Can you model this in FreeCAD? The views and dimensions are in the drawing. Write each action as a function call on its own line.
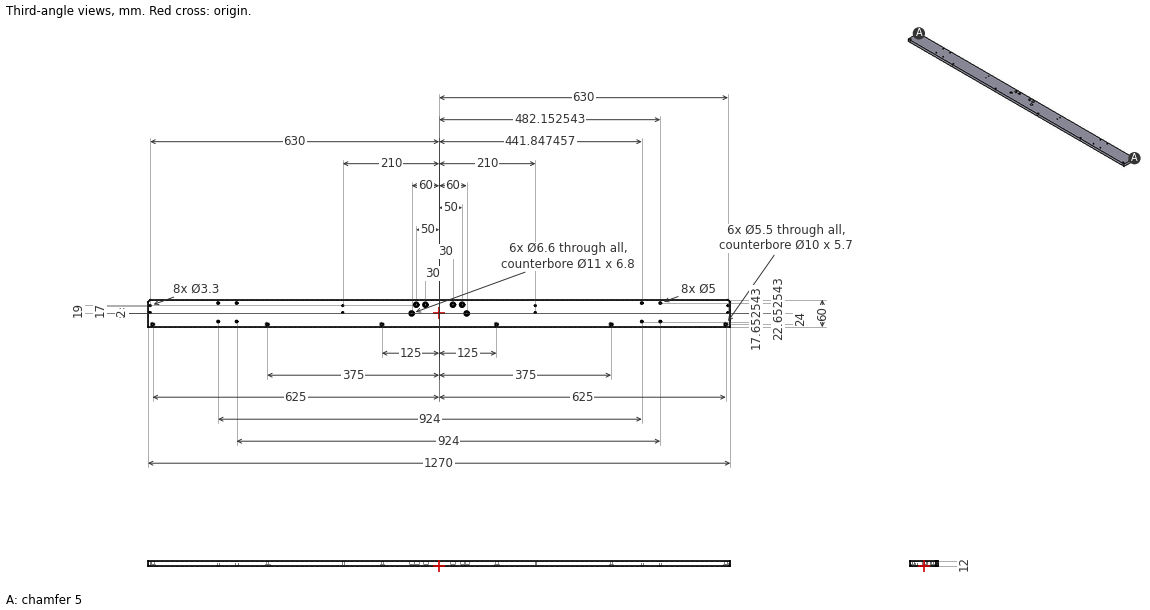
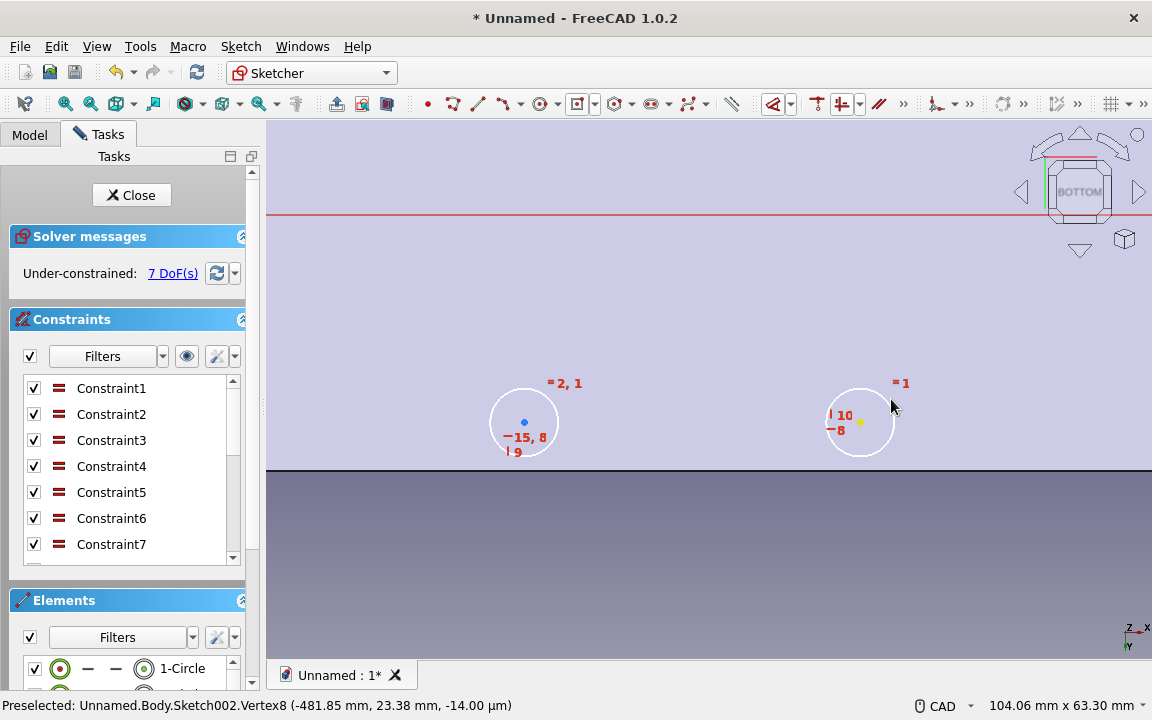
click(884, 399)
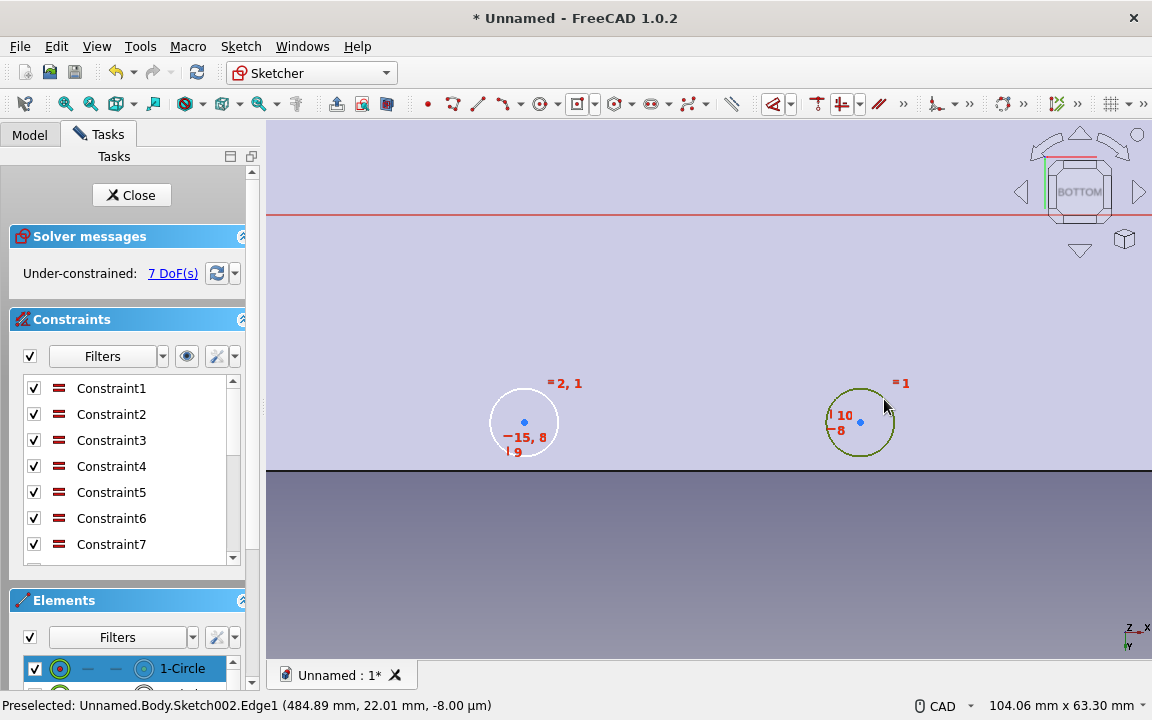
key(k)
key(o)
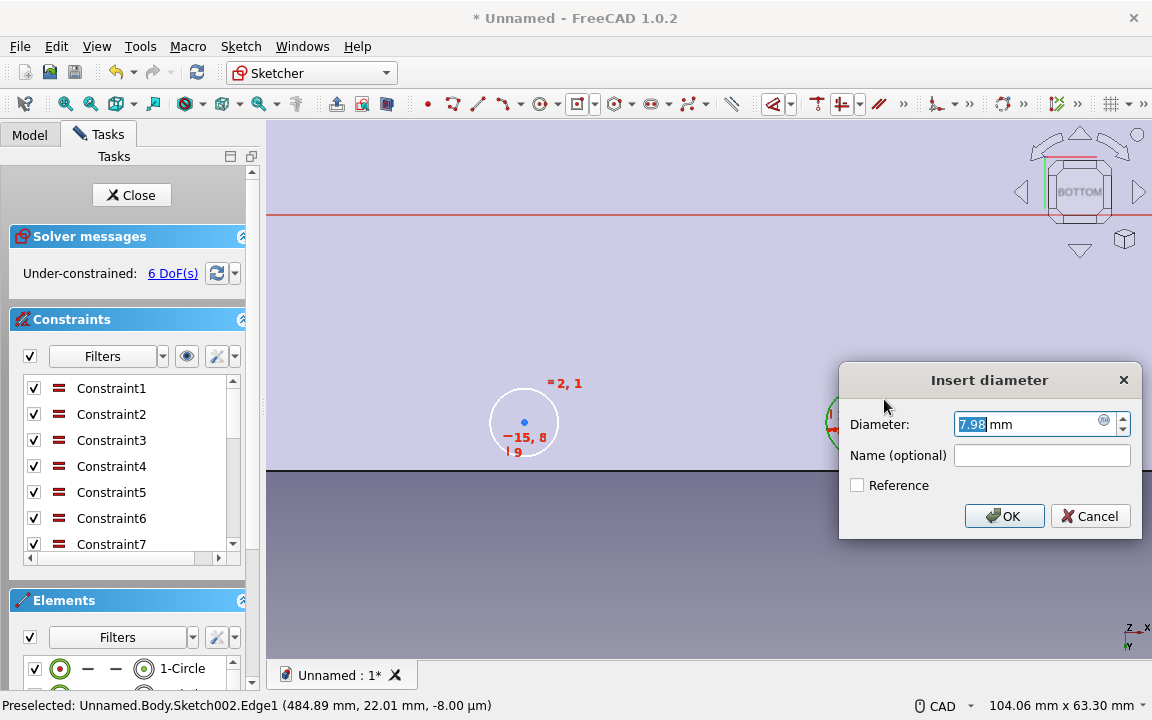
text(5)
key(Return)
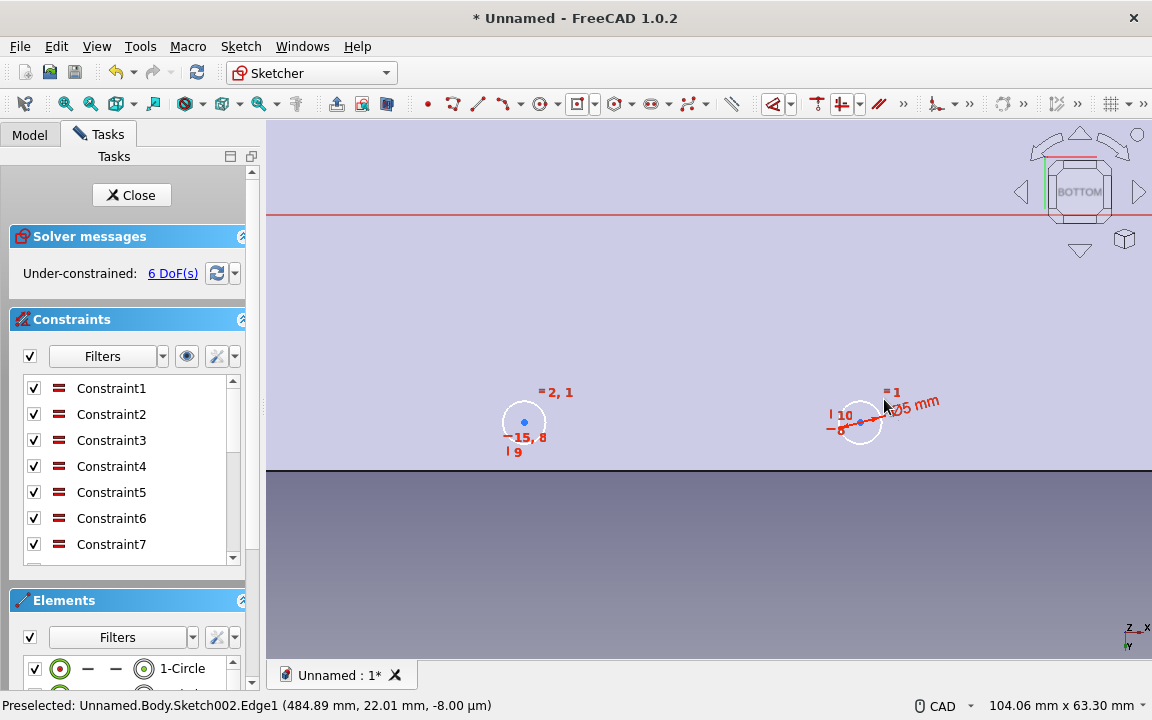
scroll(892, 399, down, 14)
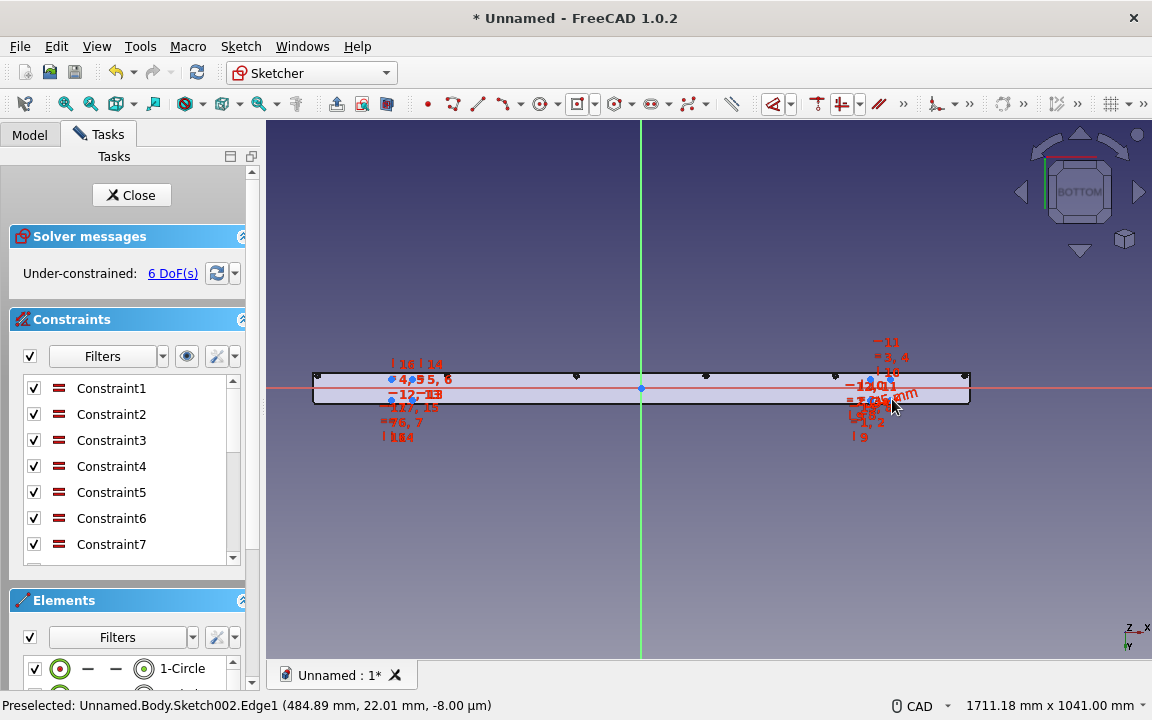
click(870, 380)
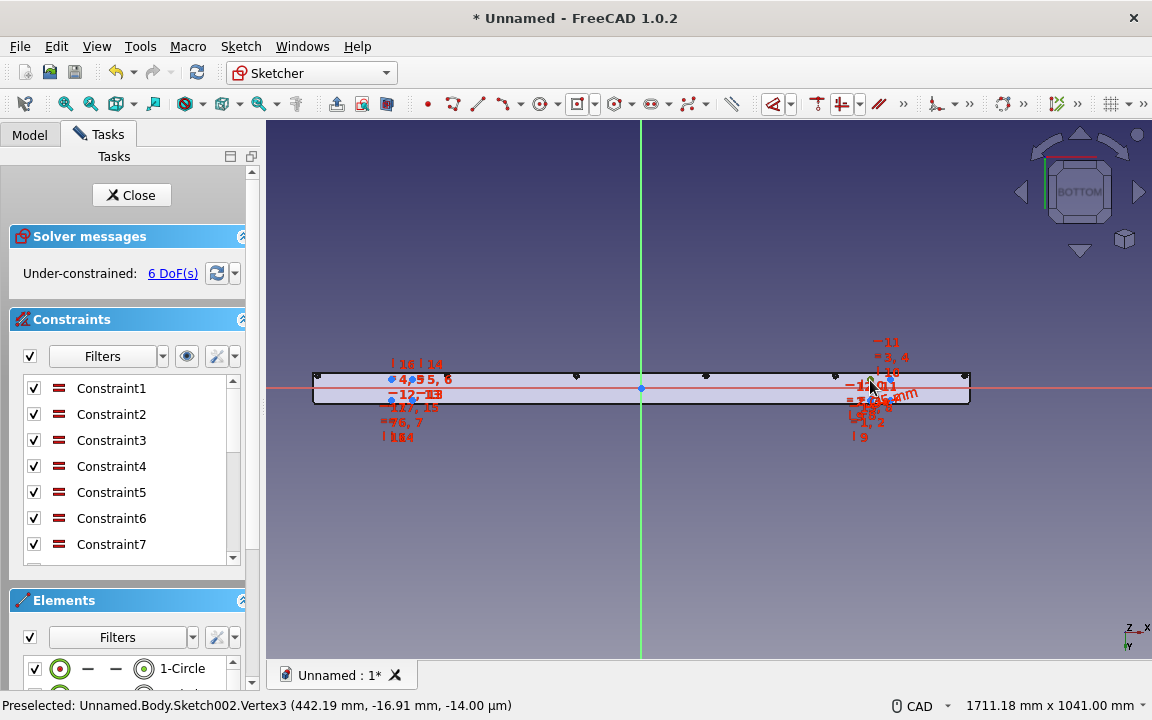
click(392, 380)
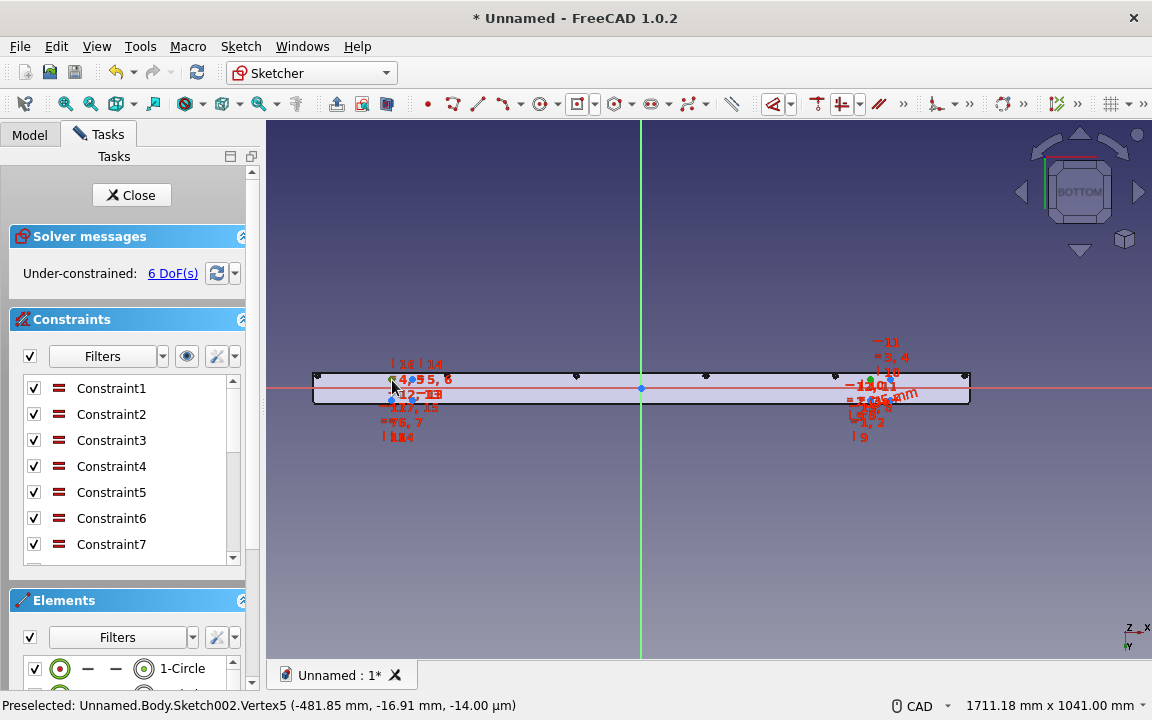
click(790, 104)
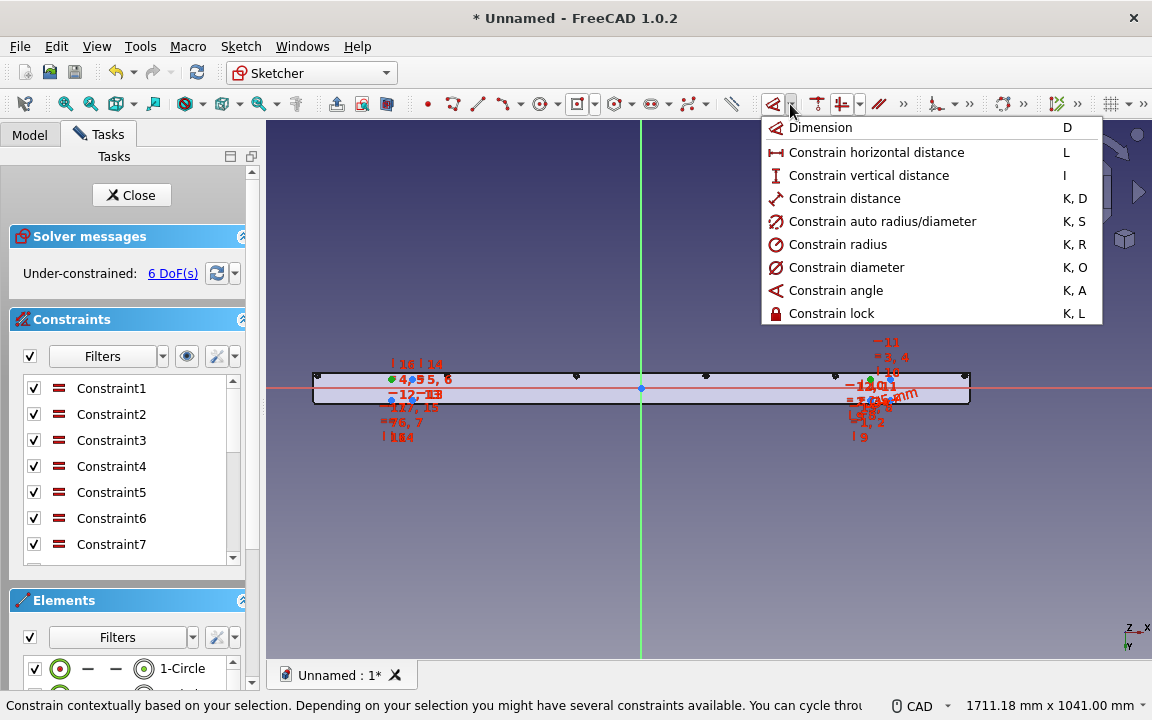
click(932, 152)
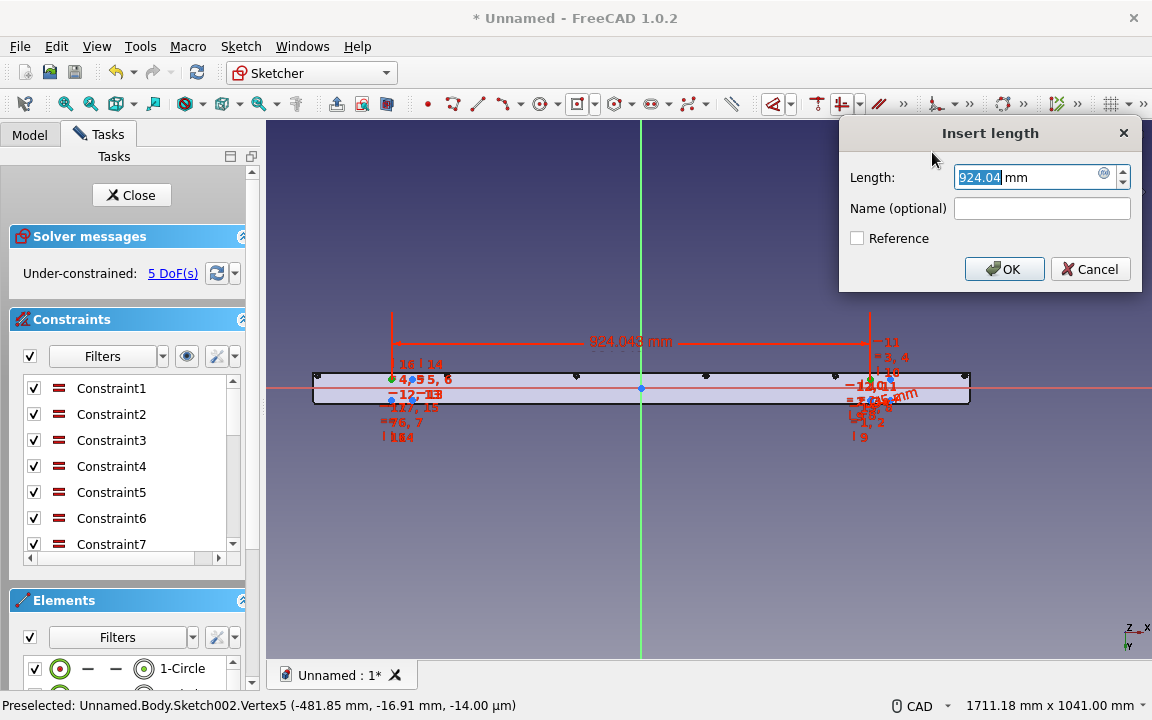
text(924)
key(Return)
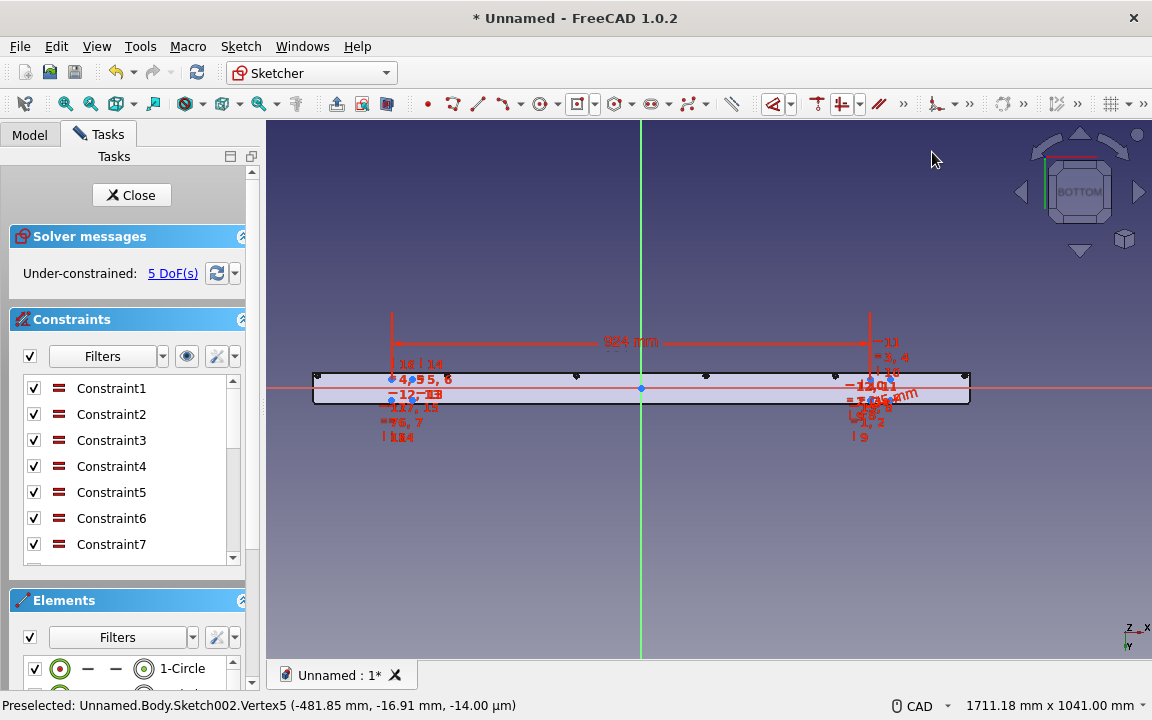
click(891, 380)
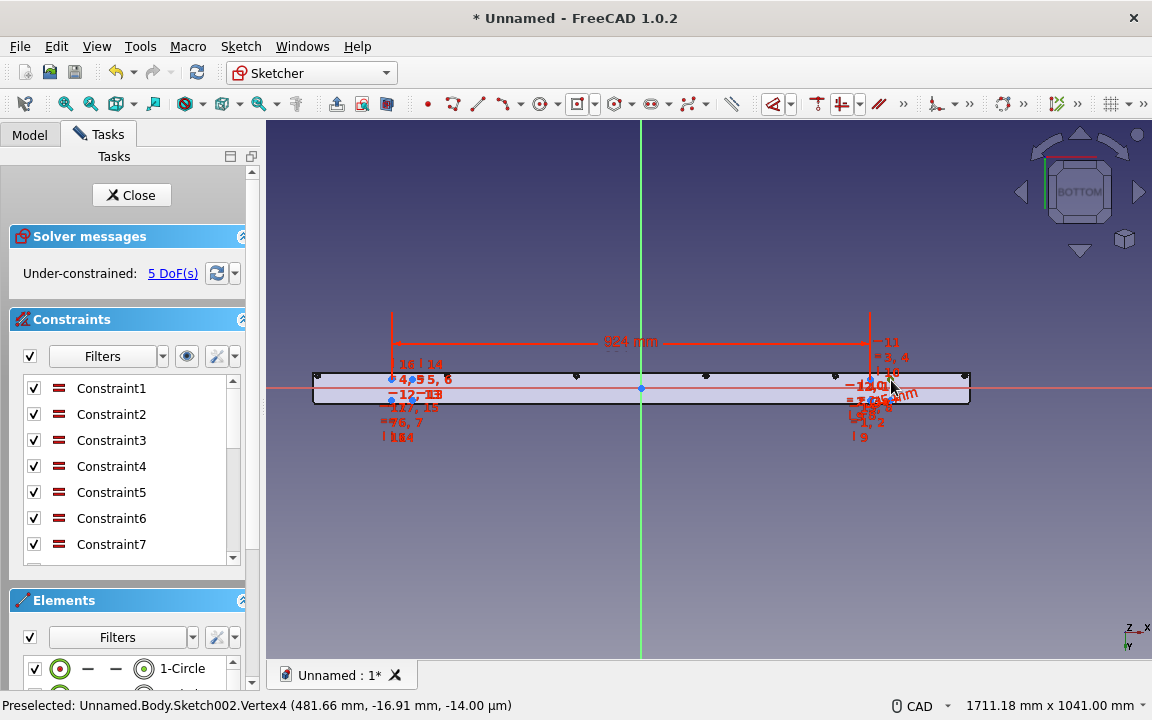
click(412, 380)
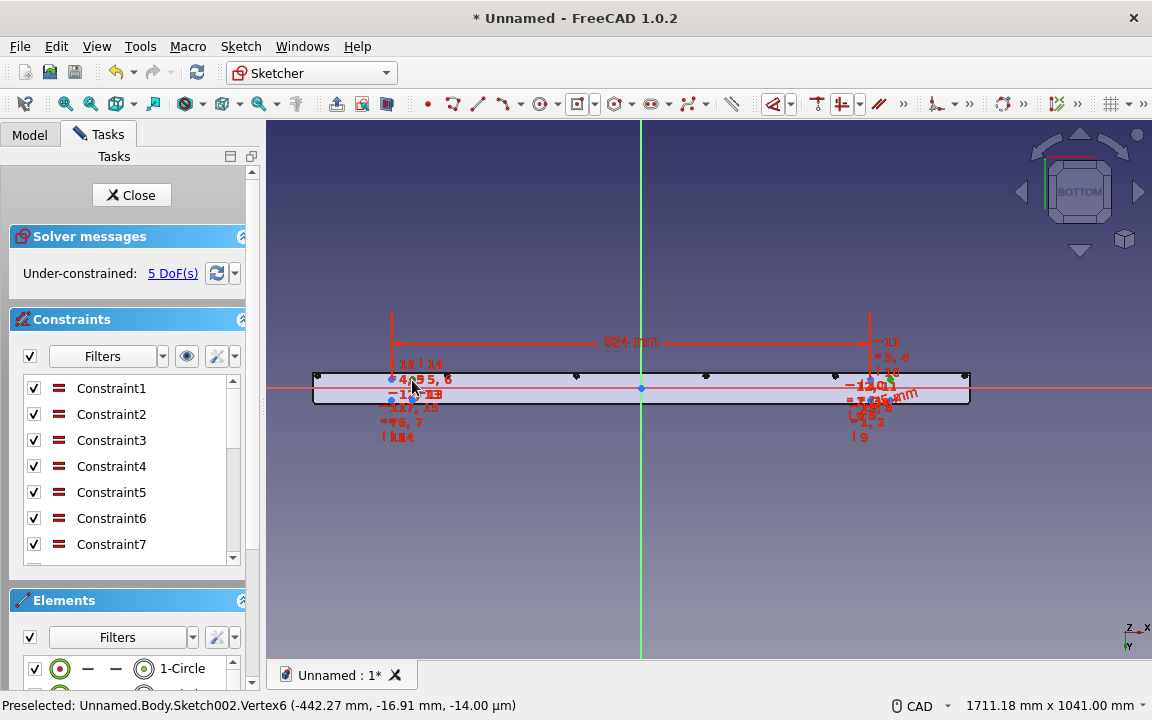
key(l)